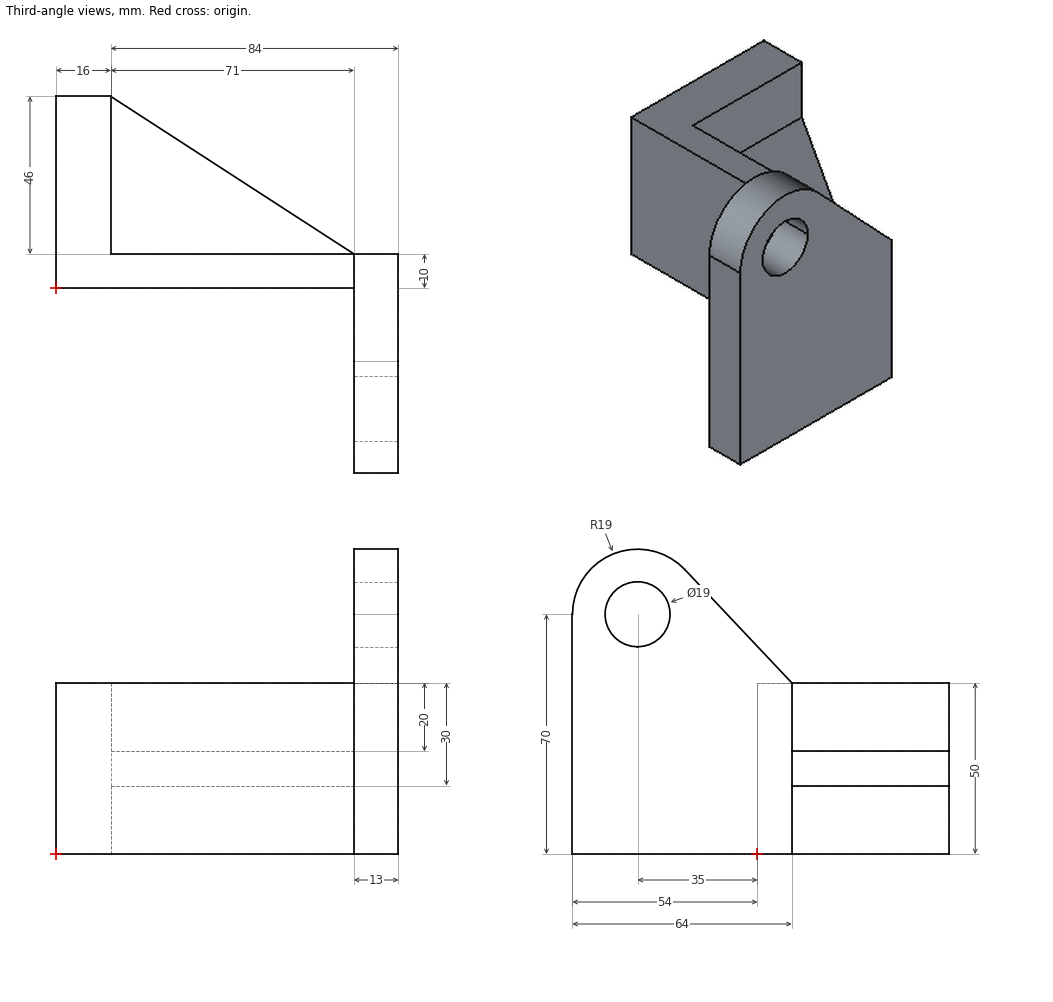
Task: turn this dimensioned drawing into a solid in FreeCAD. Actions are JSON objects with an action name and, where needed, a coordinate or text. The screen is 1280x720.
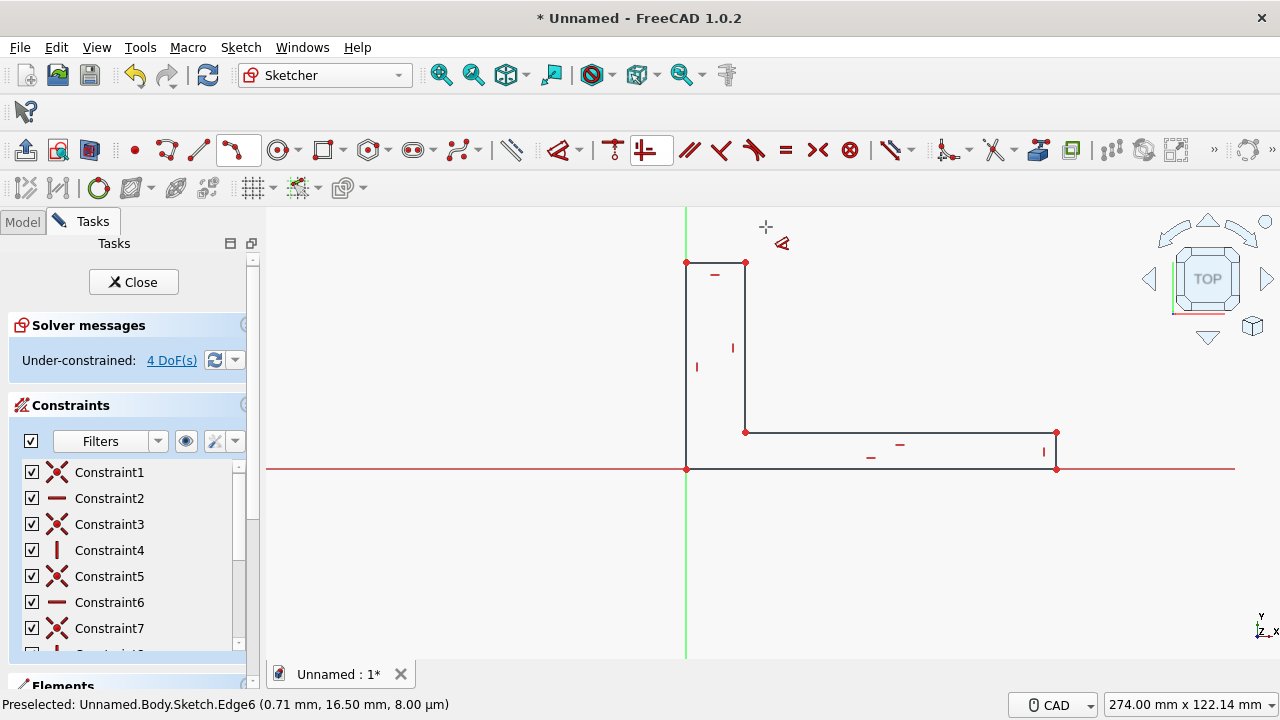
{"action": "scroll", "coordinate": [1056, 458], "scroll_direction": "up", "scroll_amount": 2}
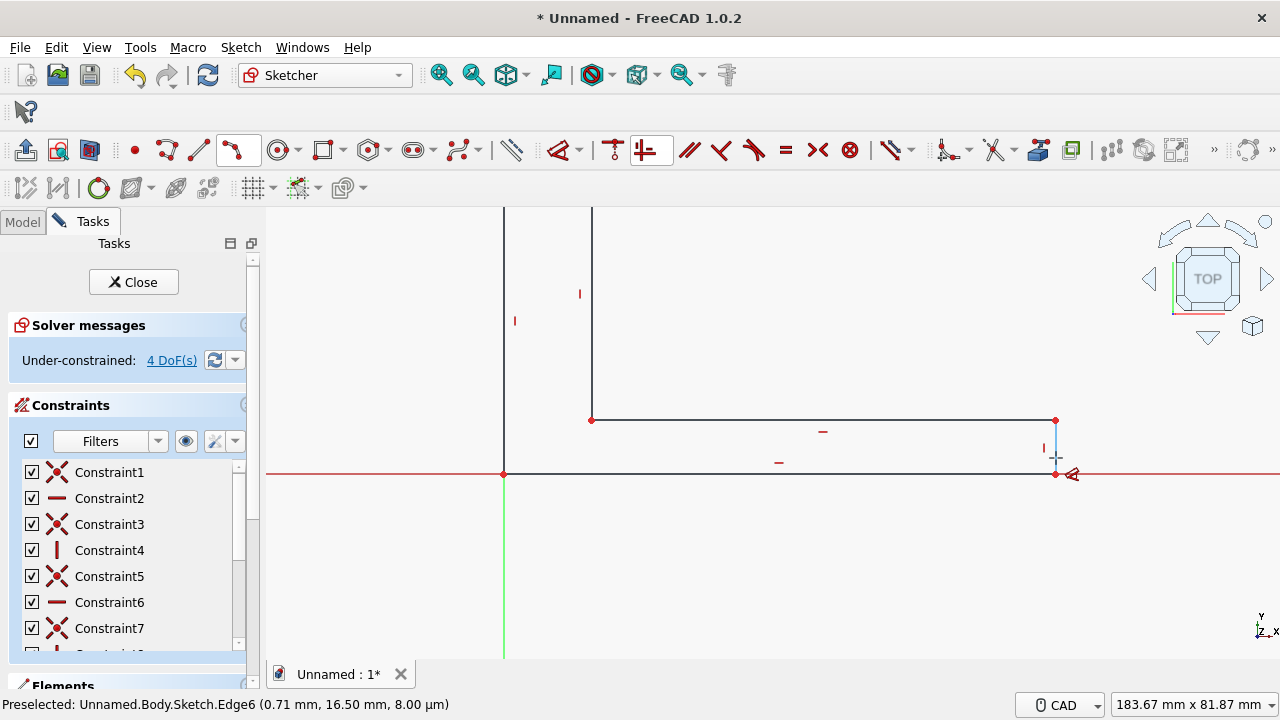
{"action": "left_click", "coordinate": [1056, 458]}
{"action": "left_click", "coordinate": [1090, 447]}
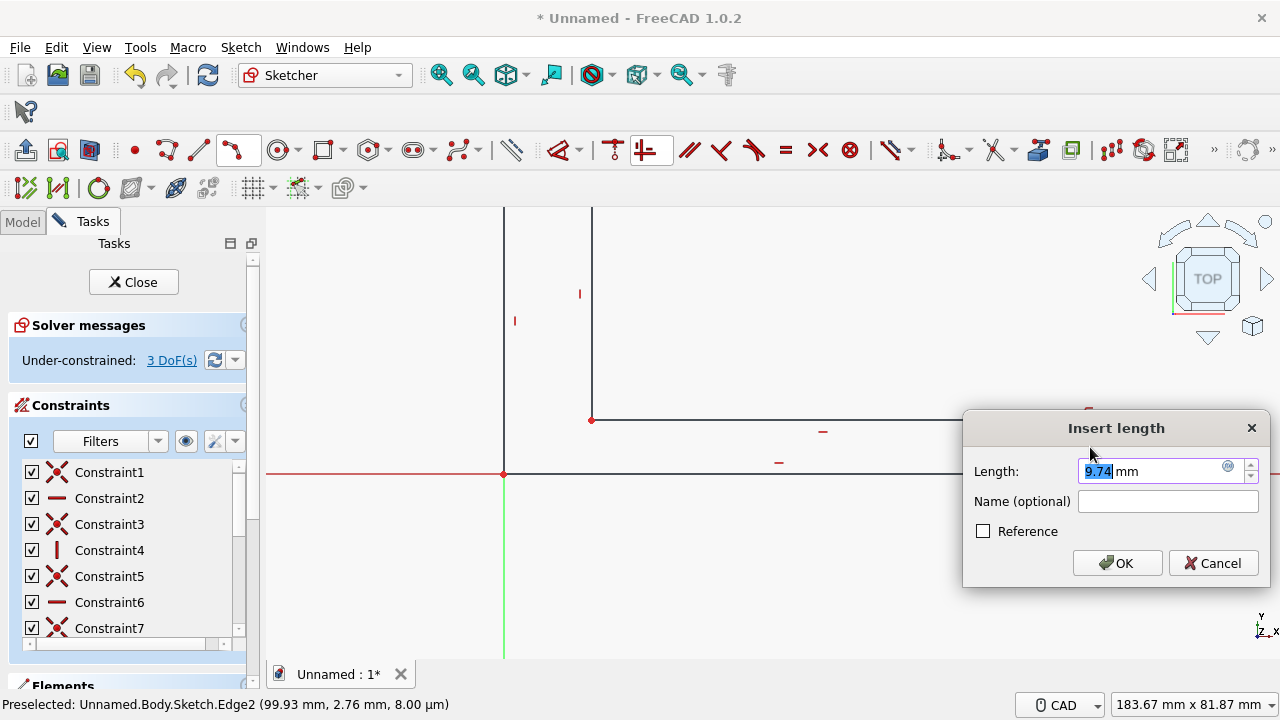
{"action": "type", "text": "10"}
{"action": "key", "text": "Return"}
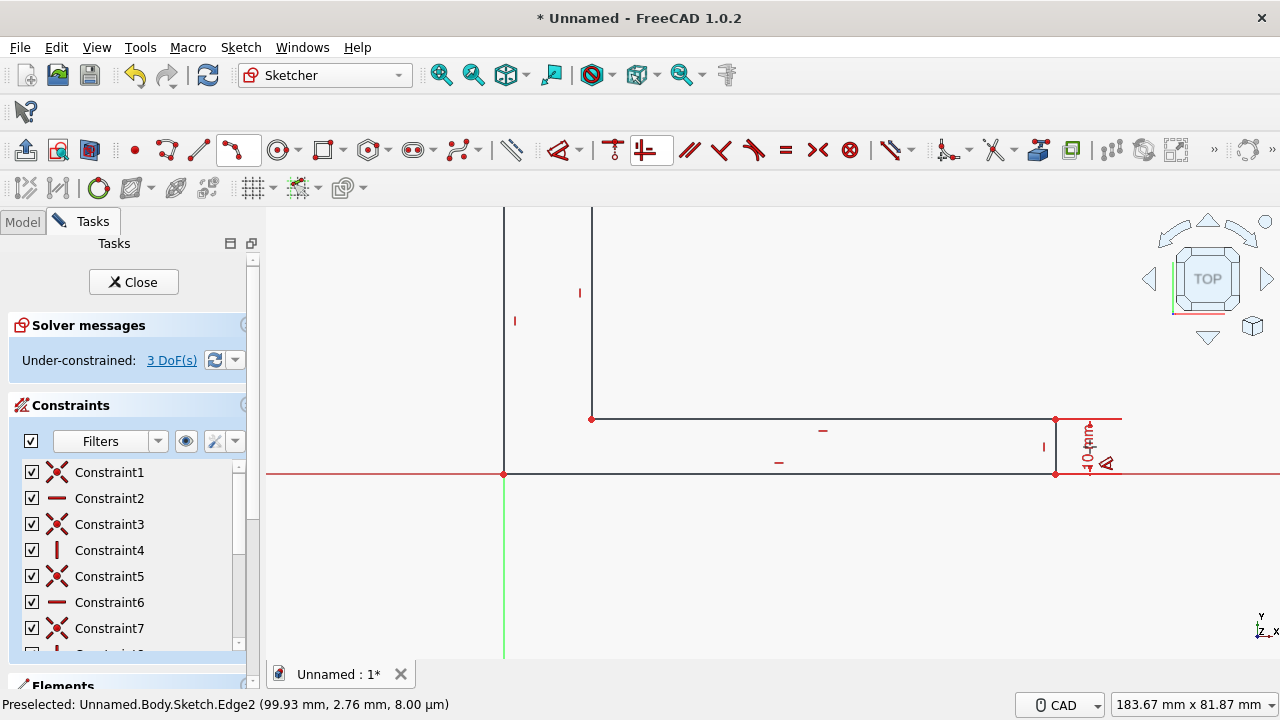
{"action": "left_click", "coordinate": [916, 419]}
{"action": "left_click", "coordinate": [824, 453]}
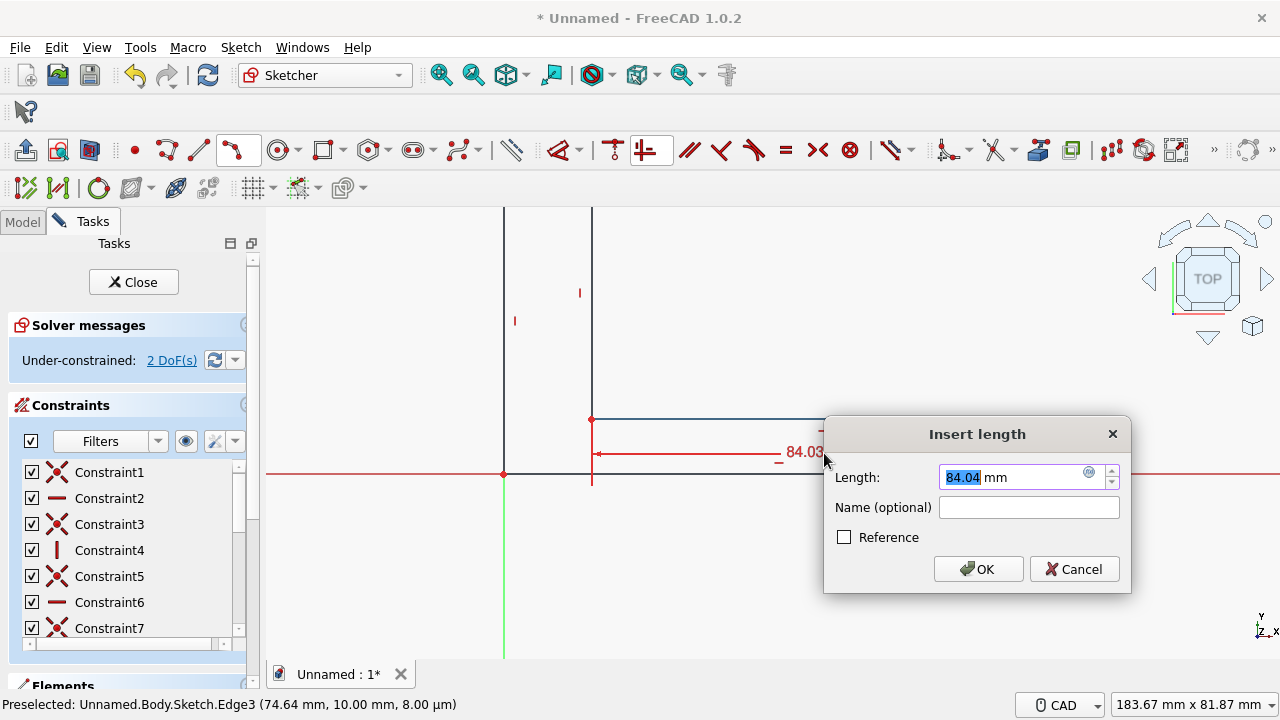
{"action": "type", "text": "84"}
{"action": "key", "text": "Return"}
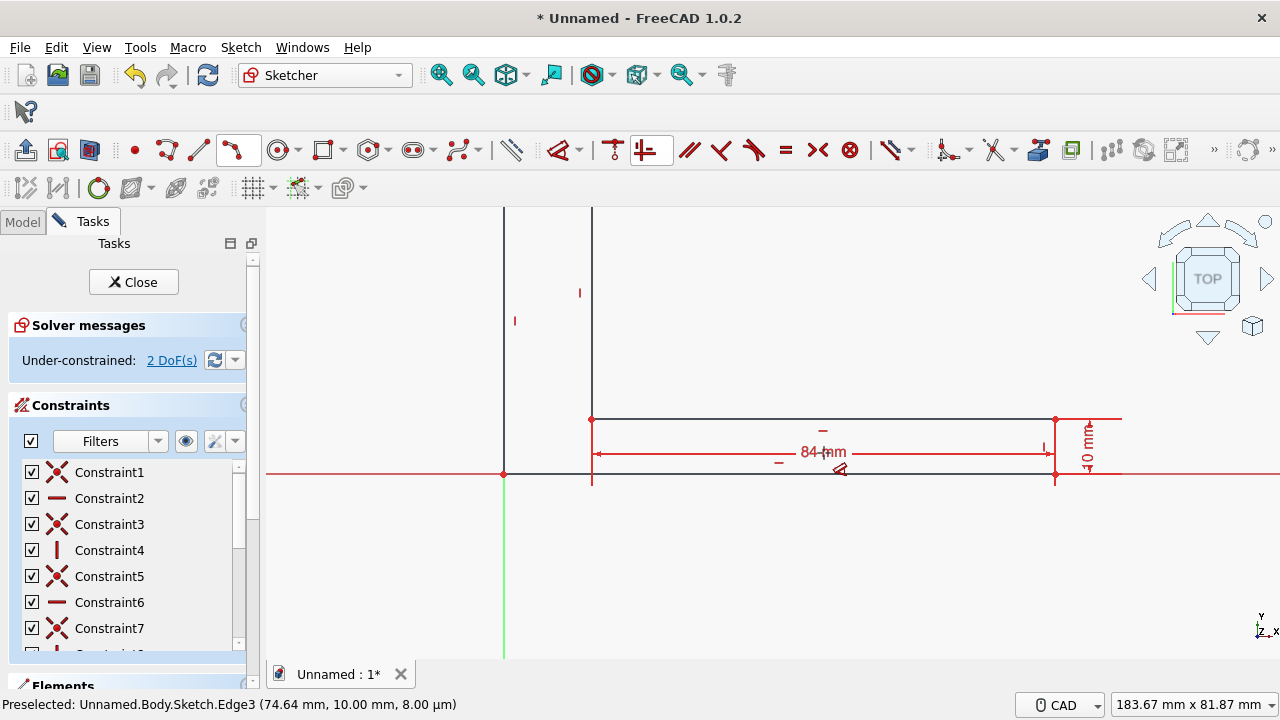
{"action": "left_click", "coordinate": [592, 343]}
{"action": "left_click", "coordinate": [558, 327]}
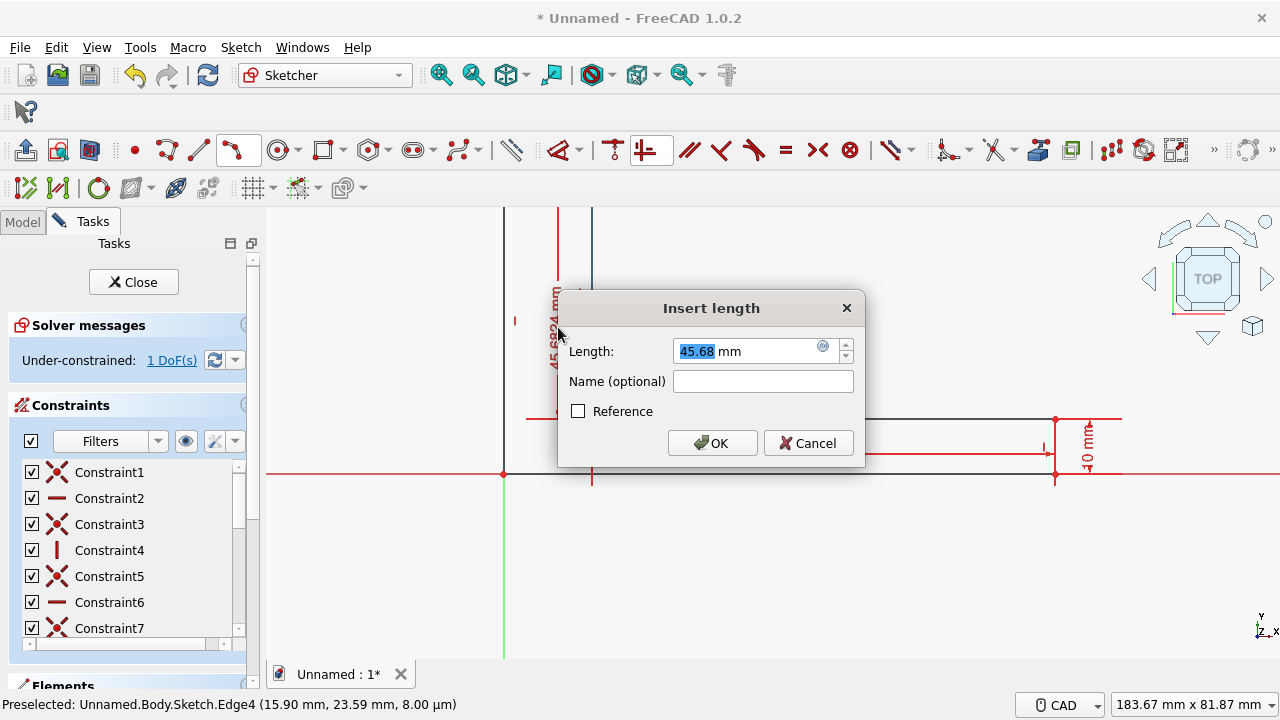
{"action": "type", "text": "46"}
{"action": "key", "text": "Return"}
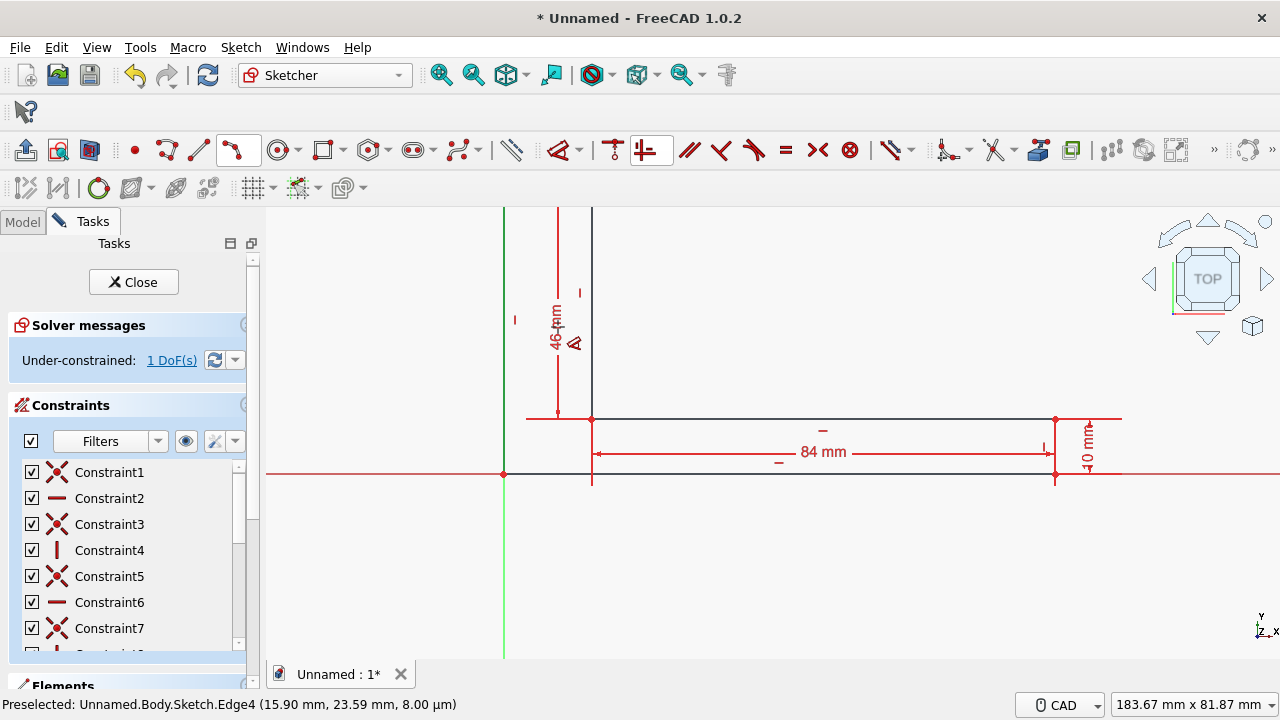
{"action": "scroll", "coordinate": [551, 631], "scroll_direction": "down", "scroll_amount": 2}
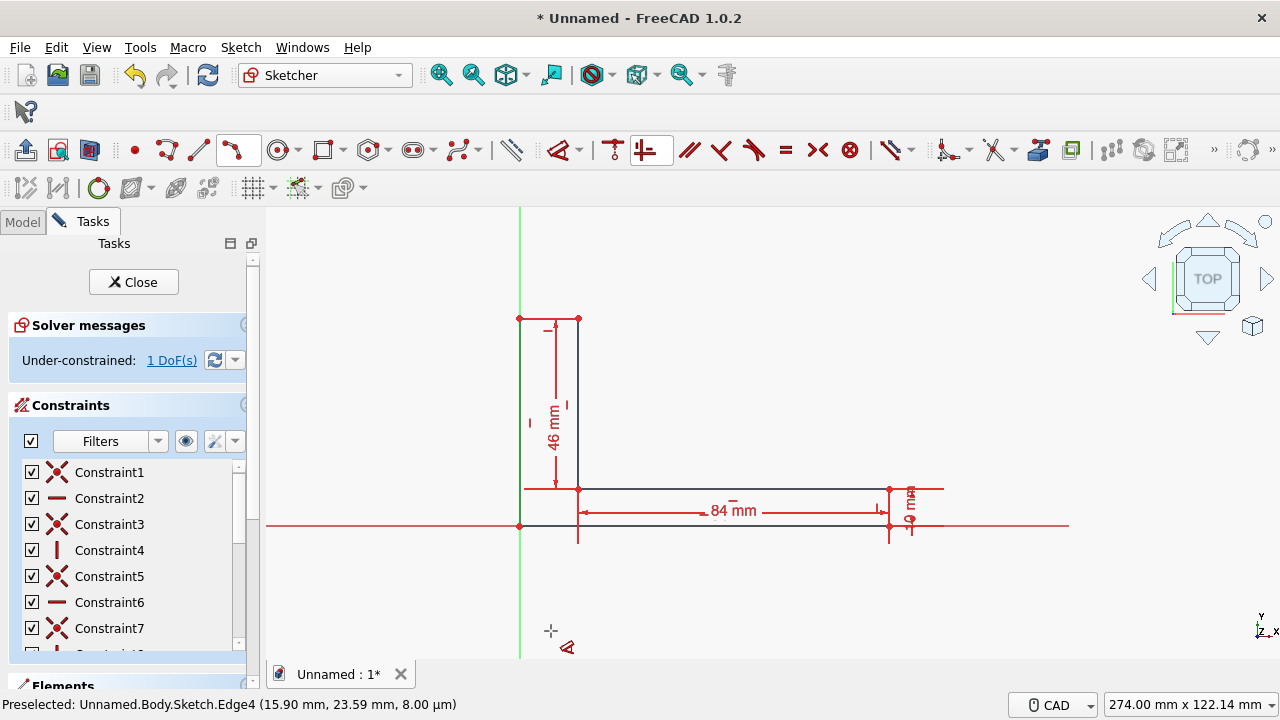
{"action": "left_click", "coordinate": [561, 319]}
{"action": "left_click", "coordinate": [549, 285]}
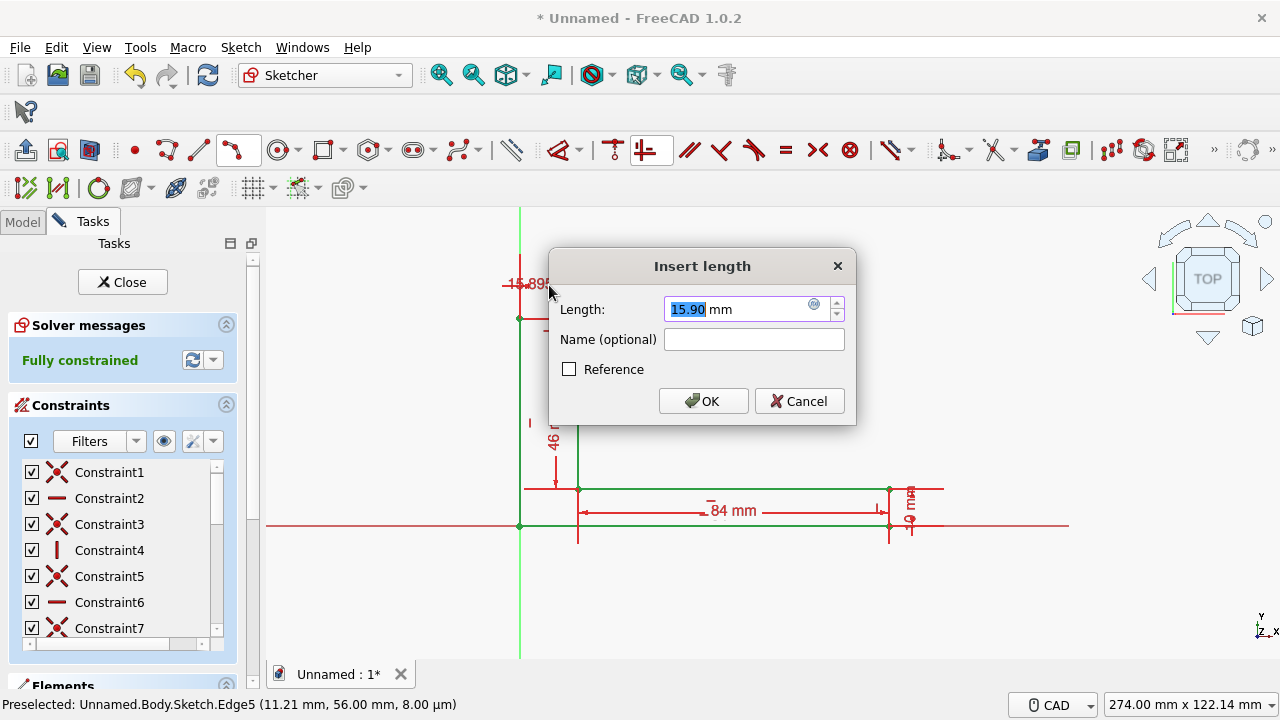
{"action": "type", "text": "16"}
{"action": "key", "text": "Return"}
{"action": "key", "text": "Escape"}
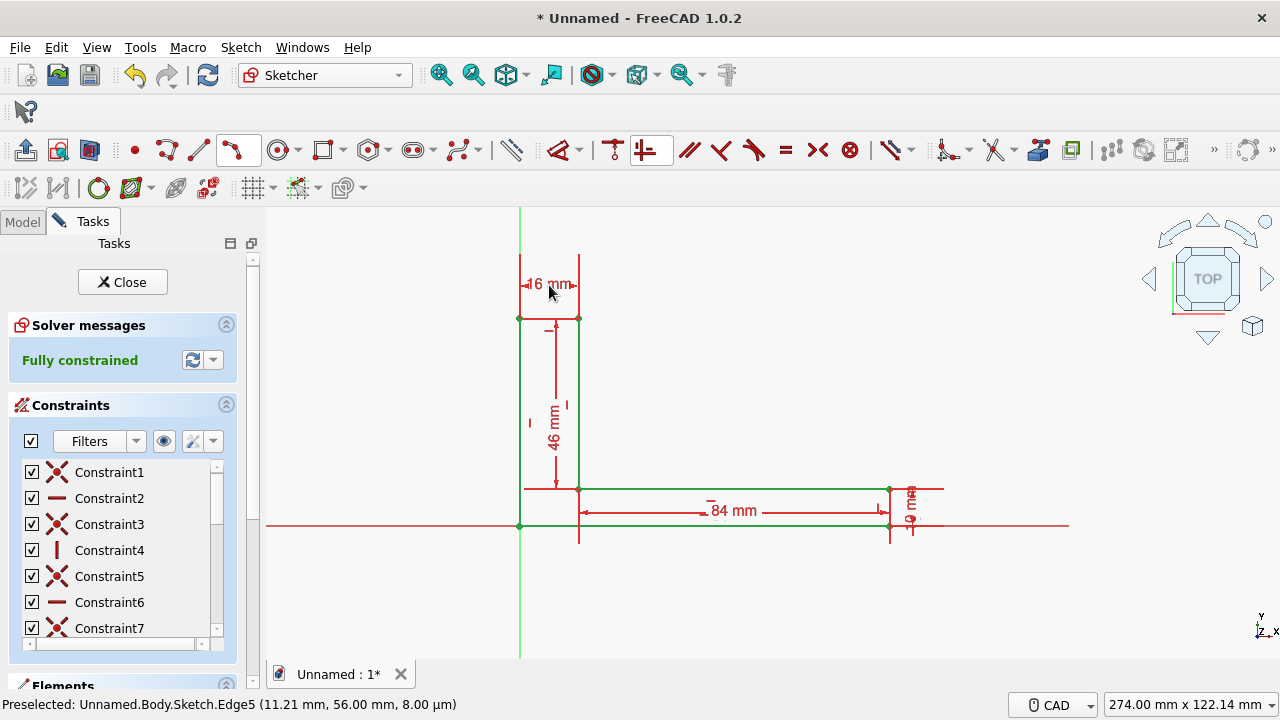
{"action": "left_click", "coordinate": [123, 282]}